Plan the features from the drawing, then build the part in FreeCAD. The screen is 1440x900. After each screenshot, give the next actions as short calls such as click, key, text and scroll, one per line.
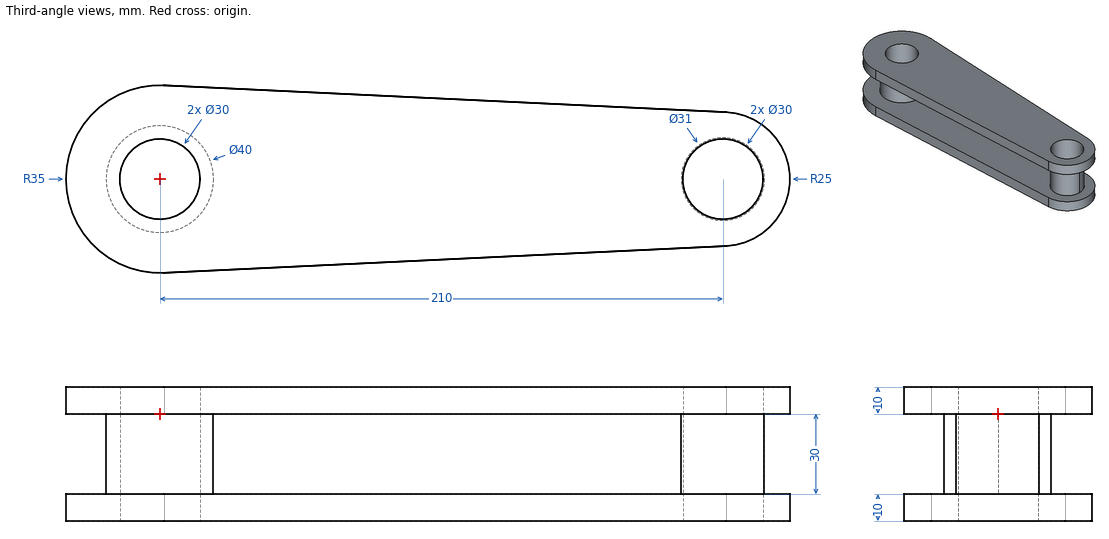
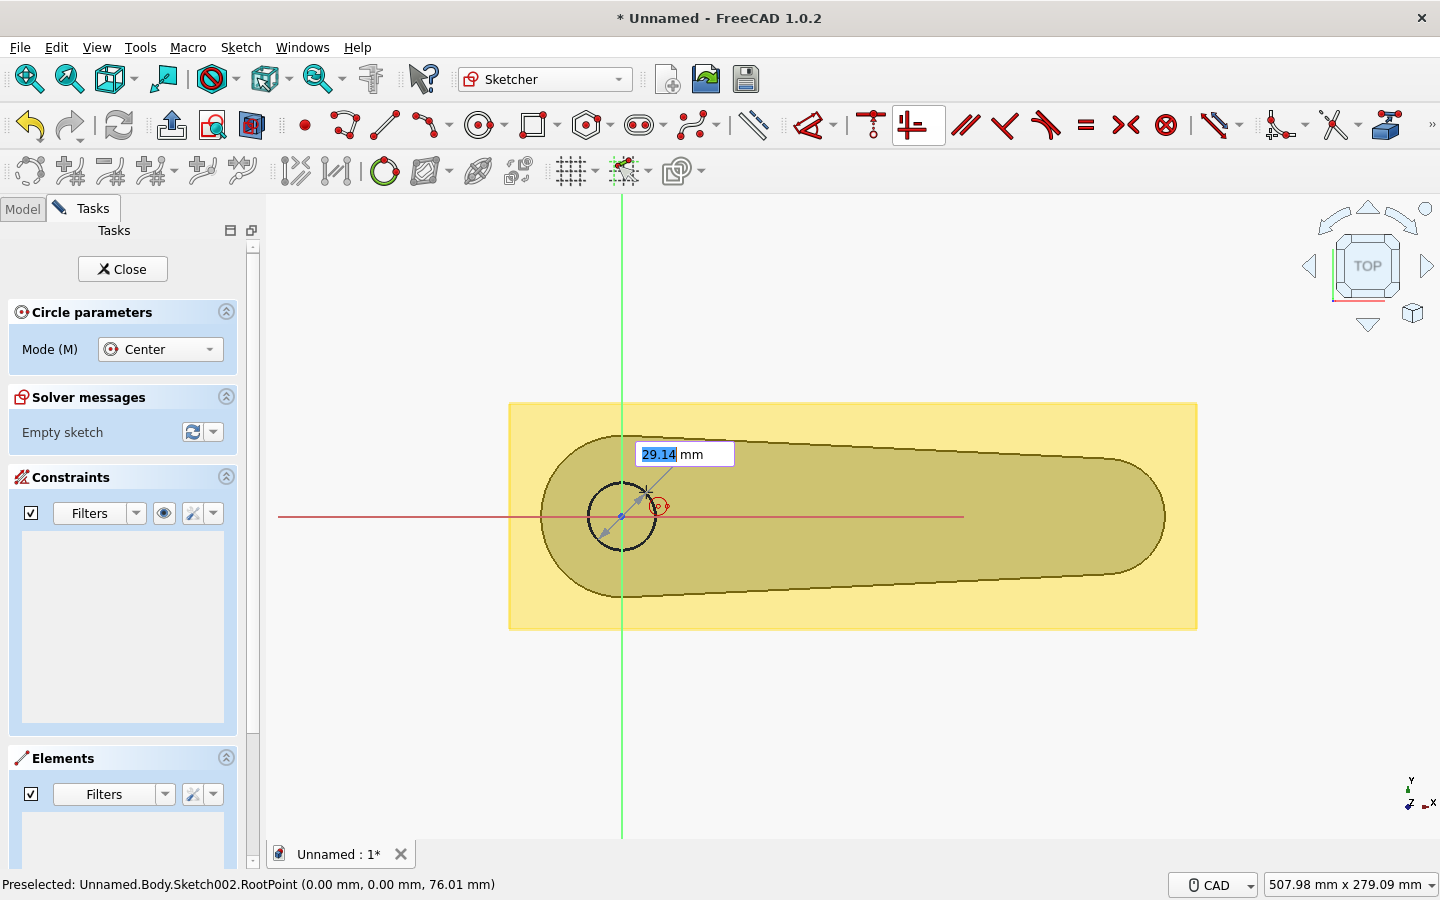
text(30)
key(Return)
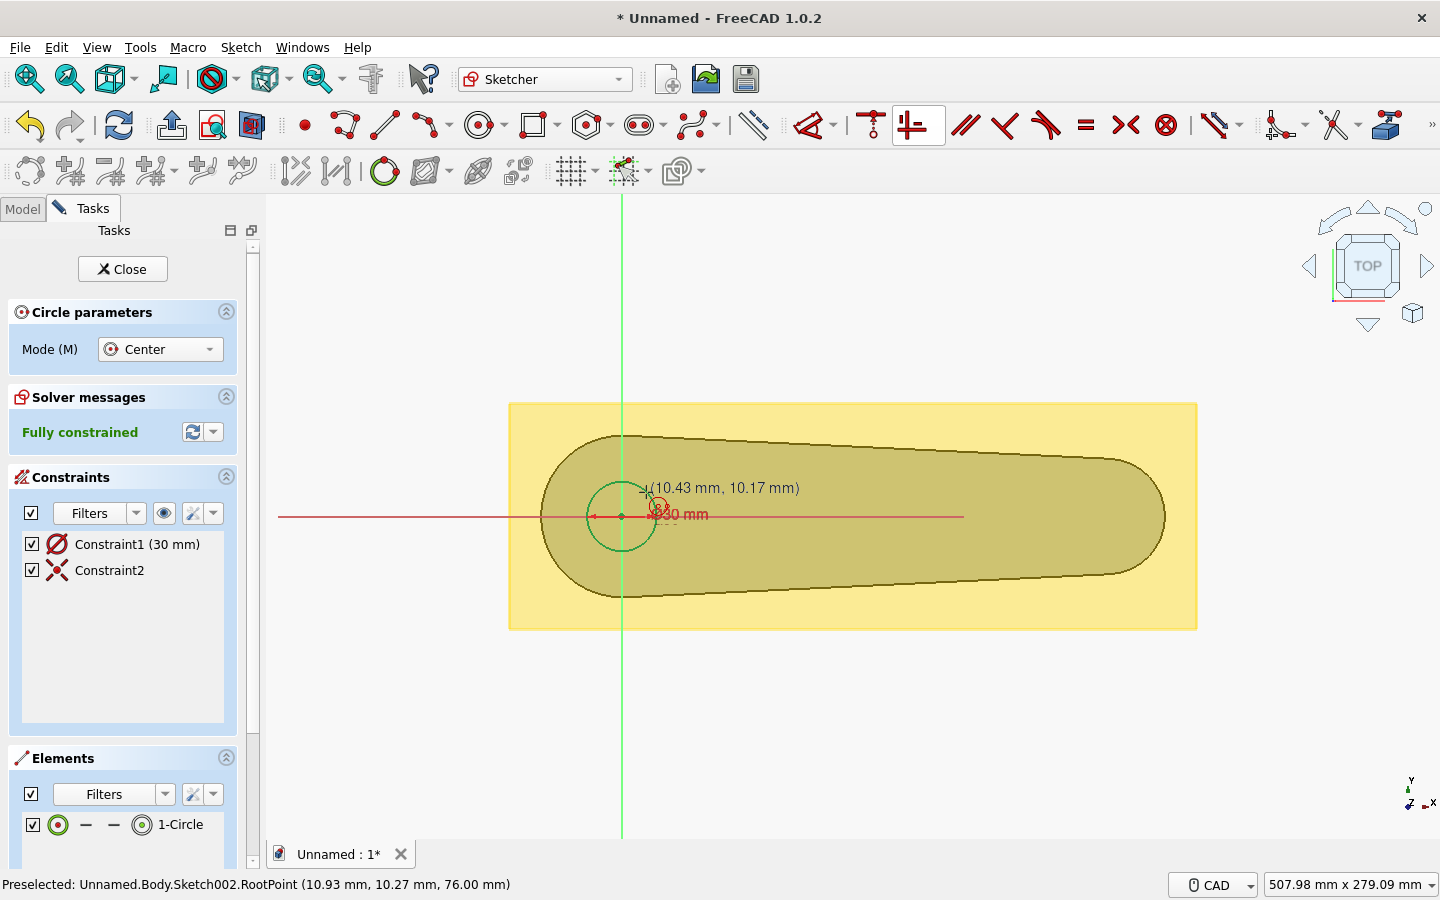
click(1107, 516)
move(1132, 492)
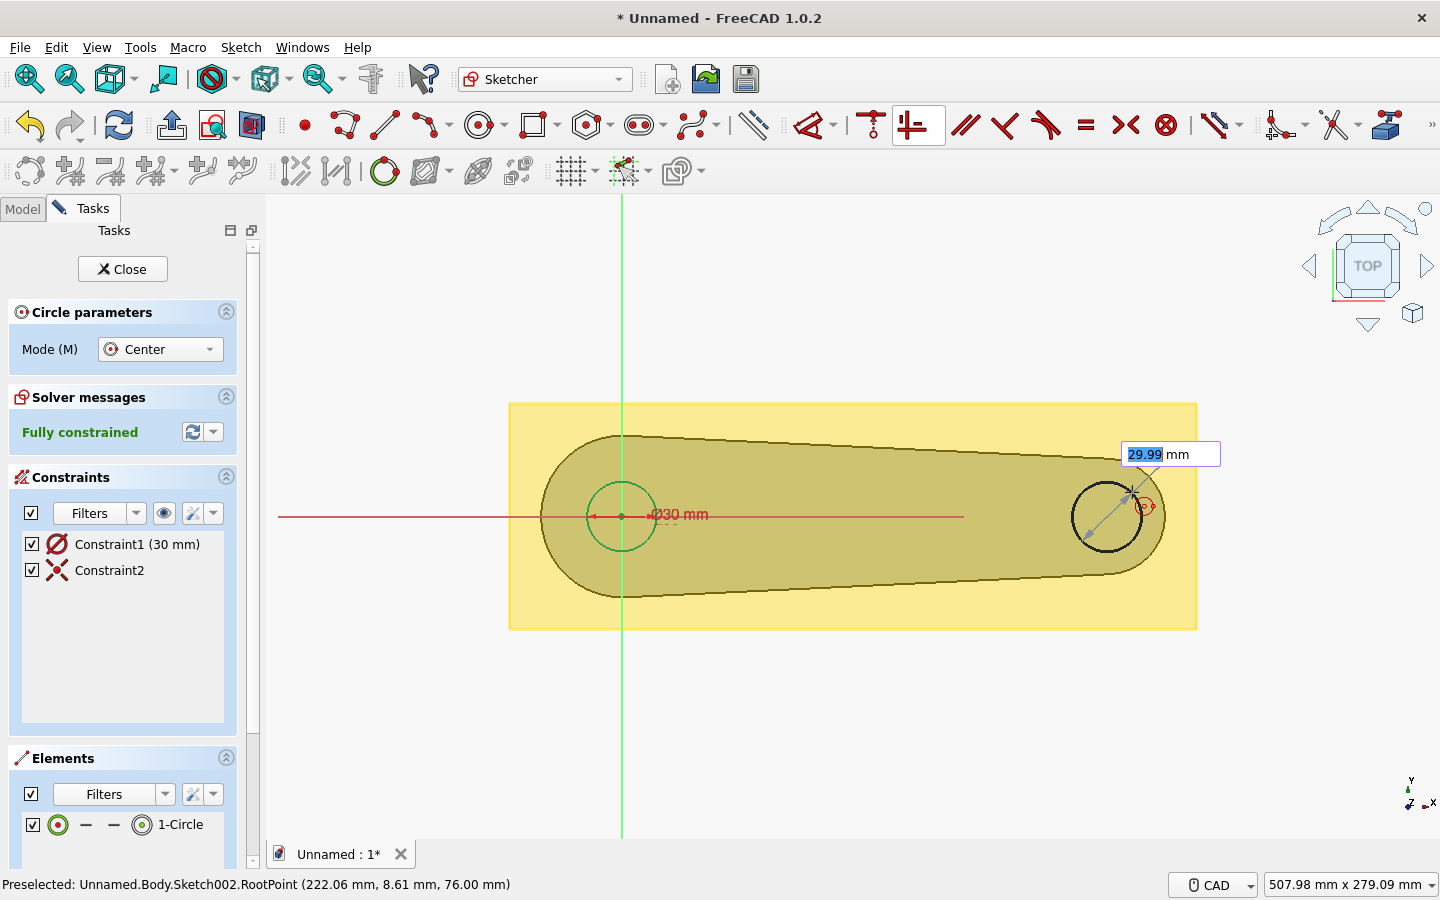
text(30)
key(Return)
key(Escape)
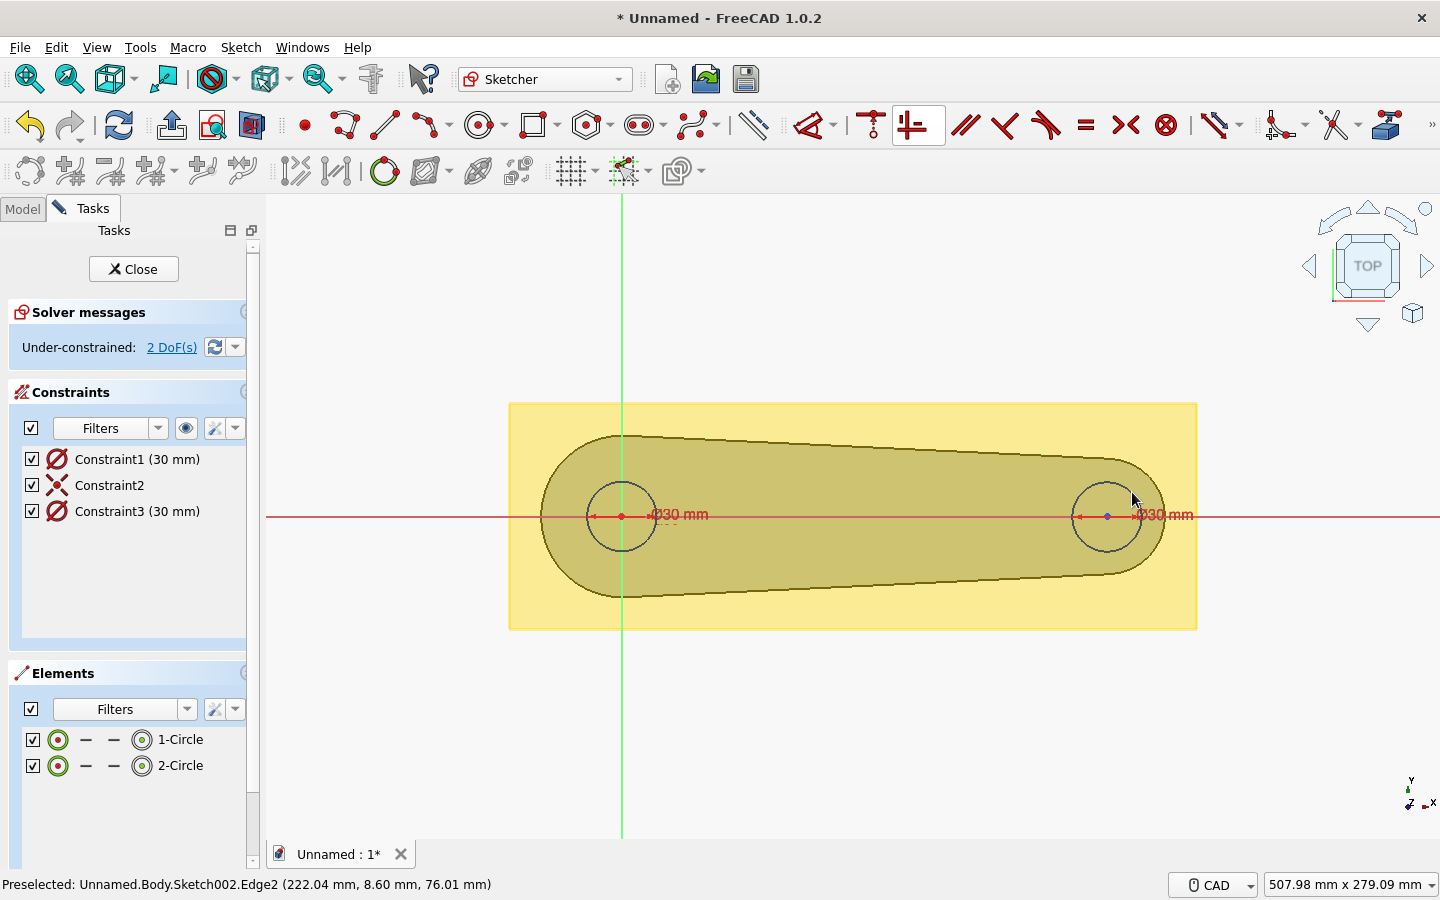
click(1107, 517)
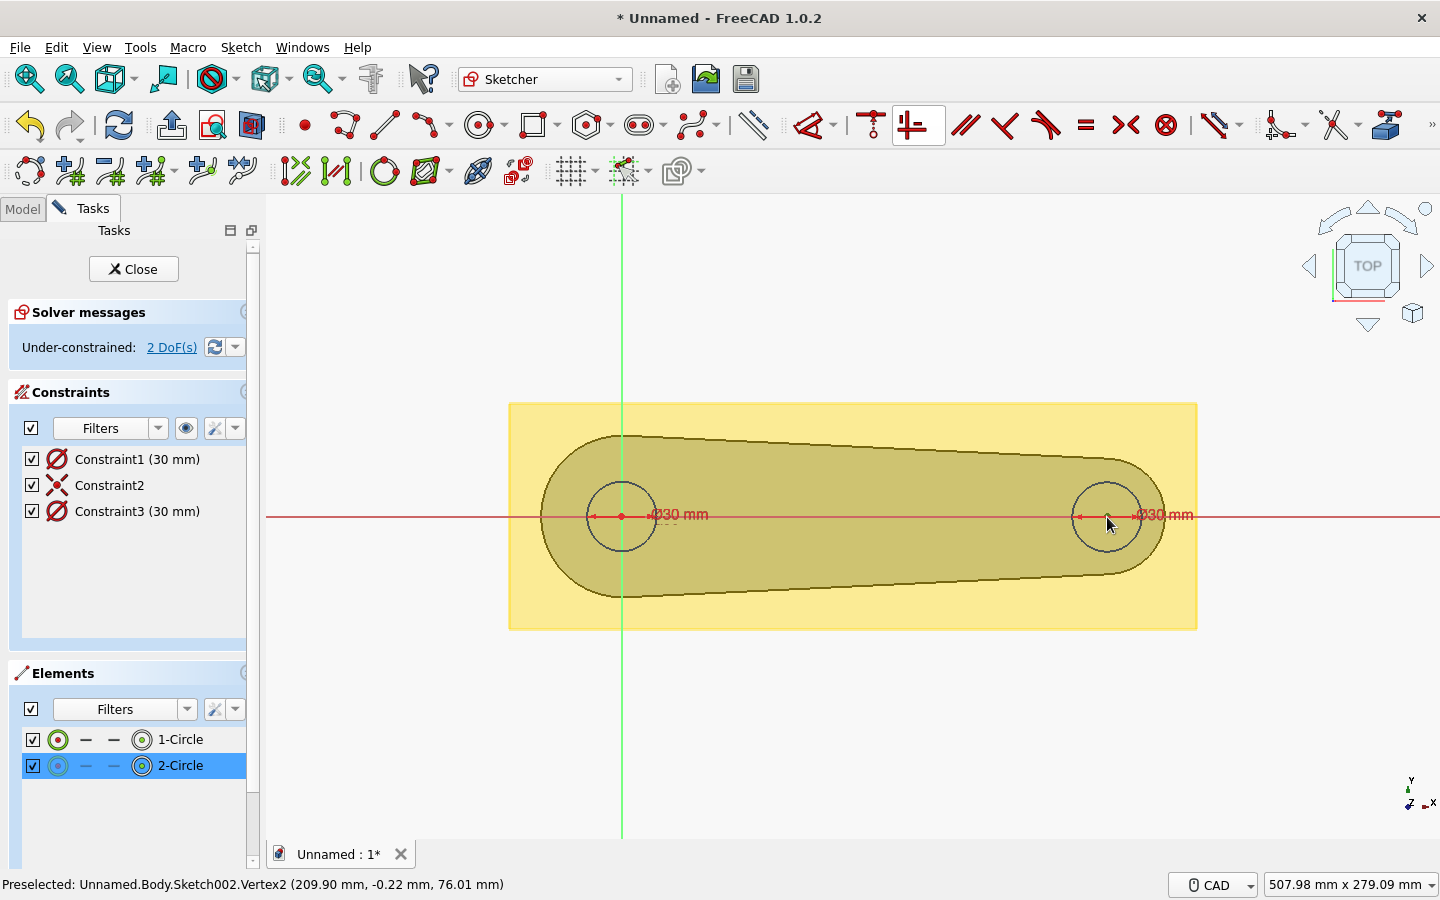
click(364, 516)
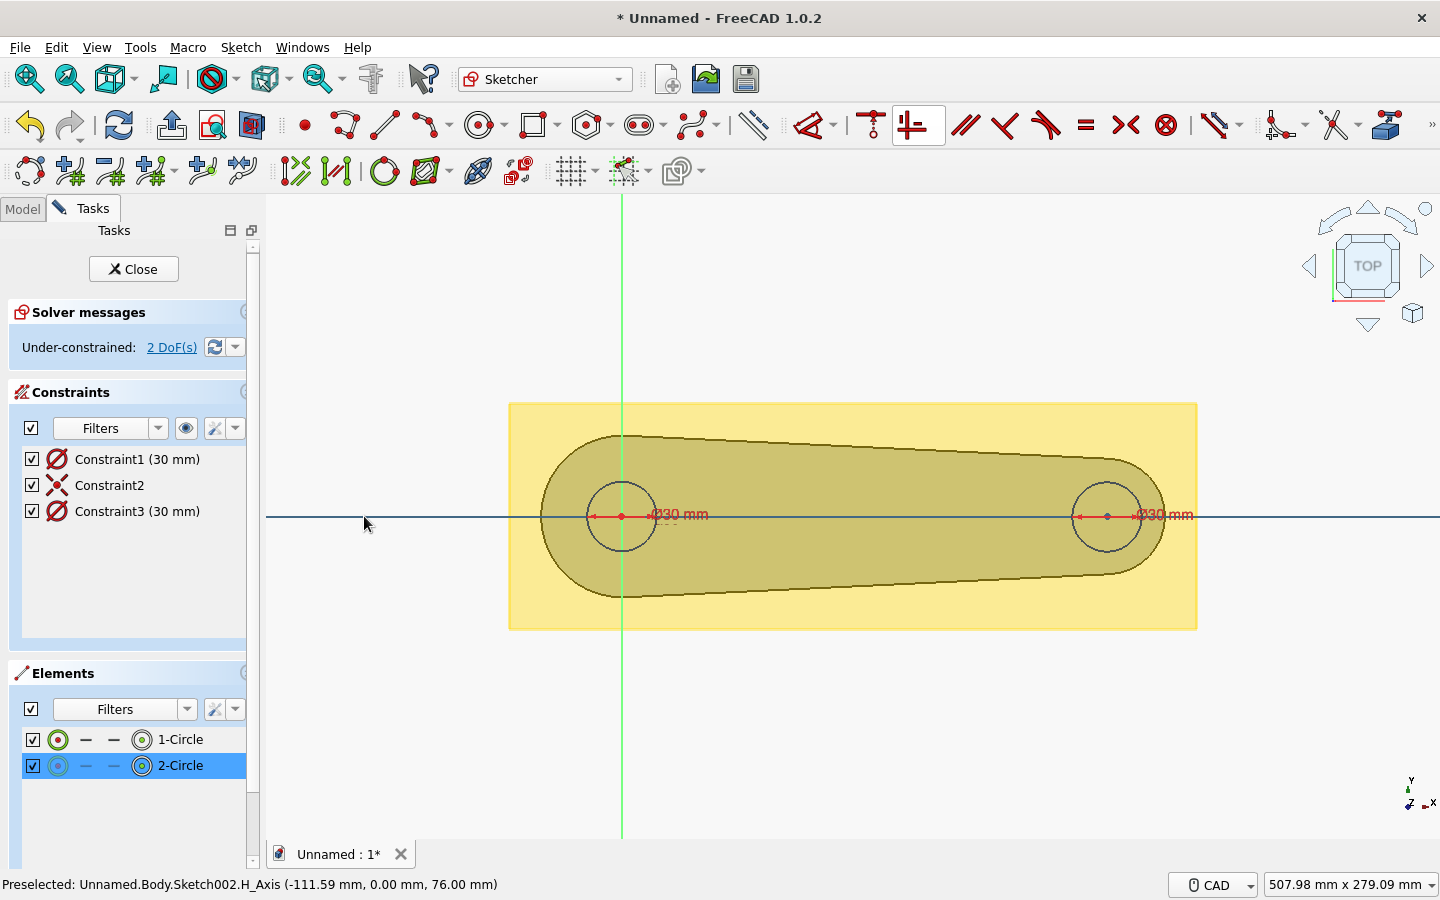
click(872, 126)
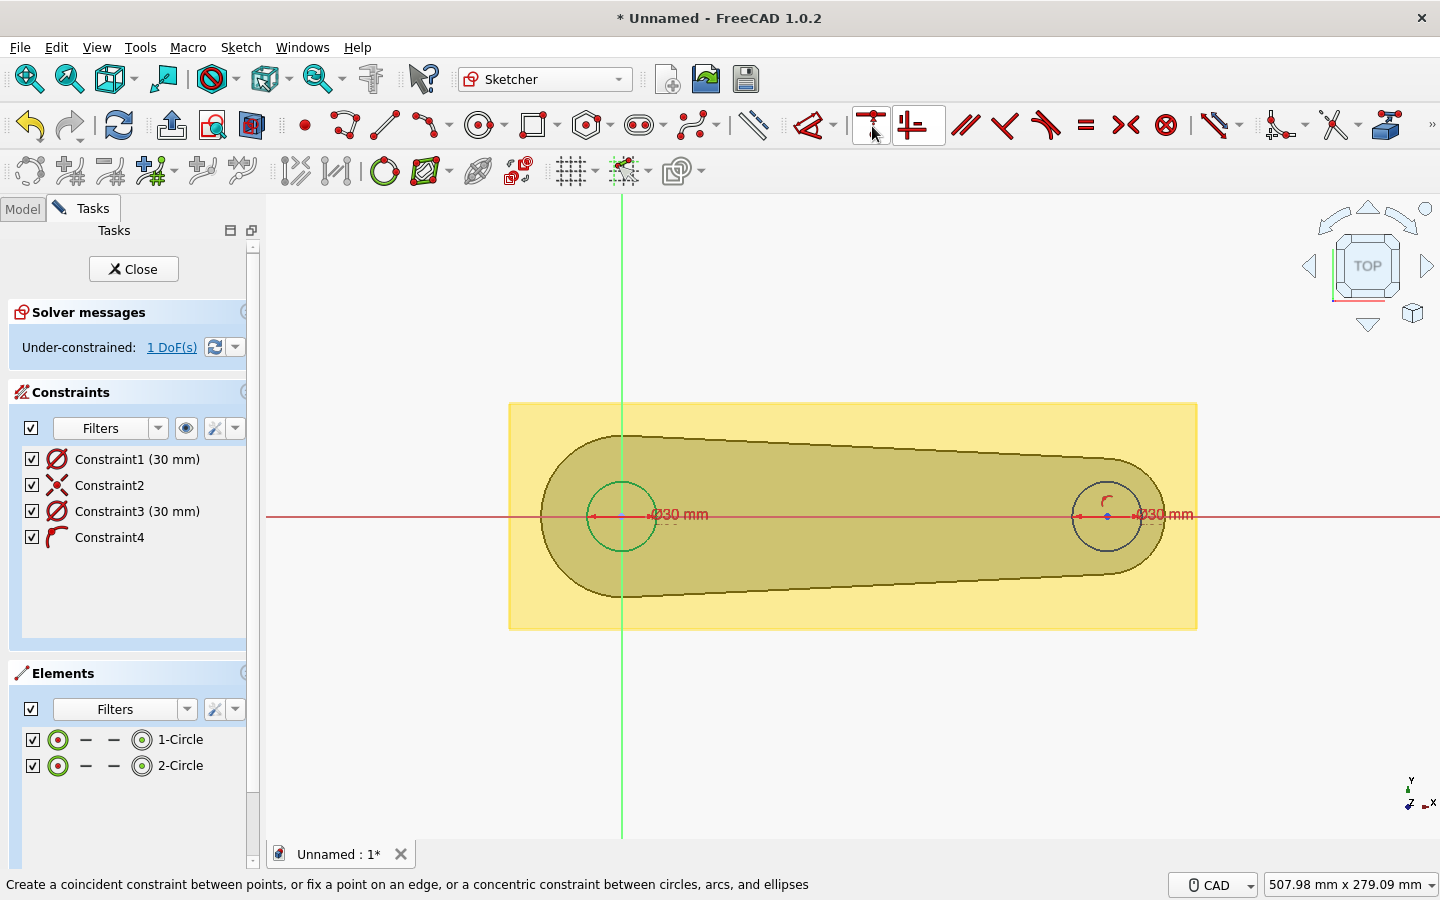
click(808, 126)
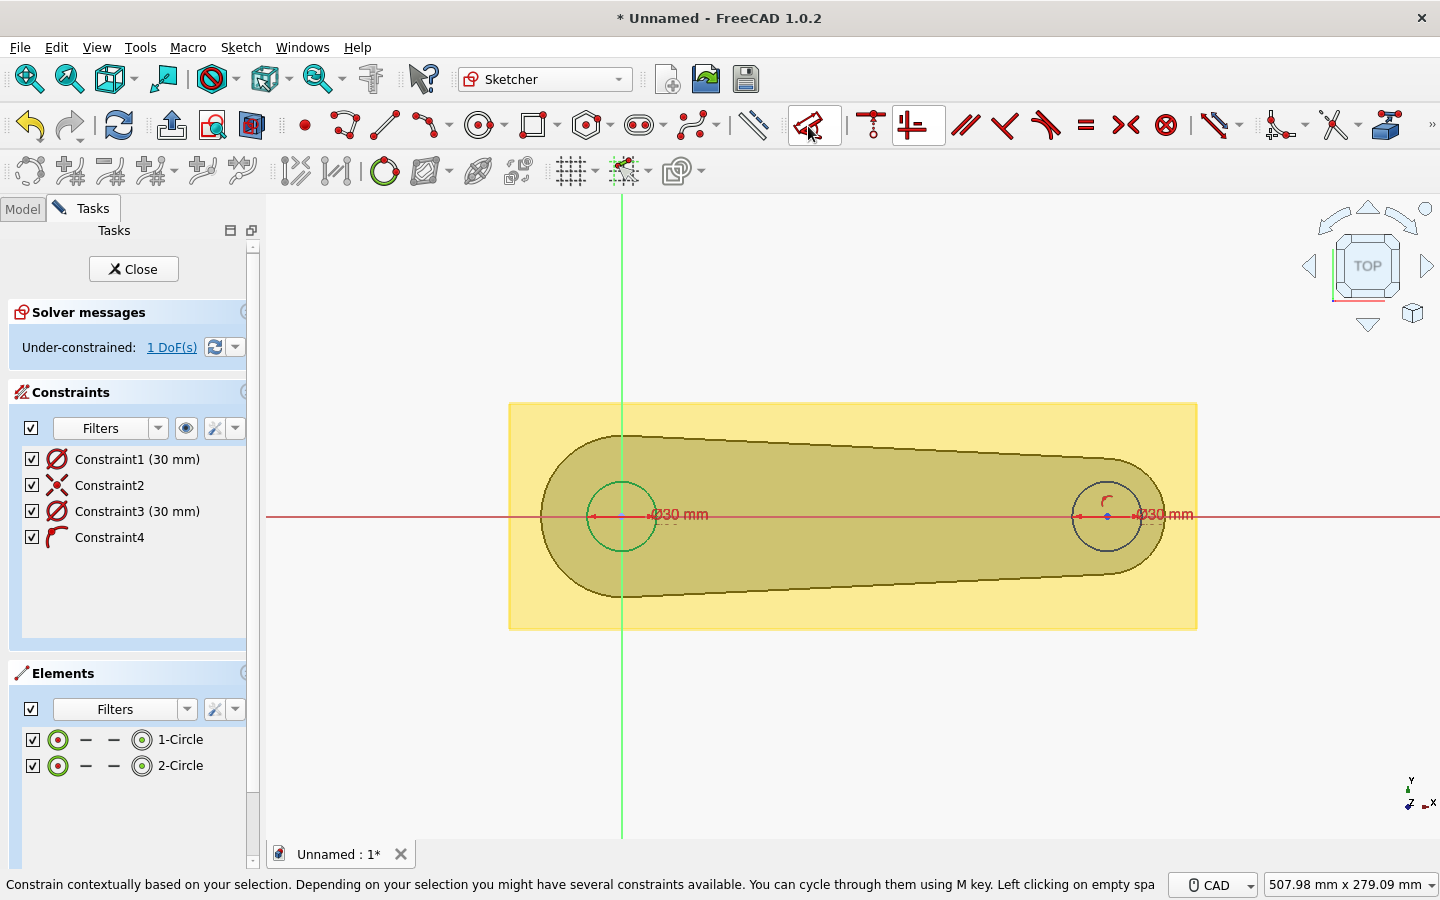
click(1107, 516)
click(864, 550)